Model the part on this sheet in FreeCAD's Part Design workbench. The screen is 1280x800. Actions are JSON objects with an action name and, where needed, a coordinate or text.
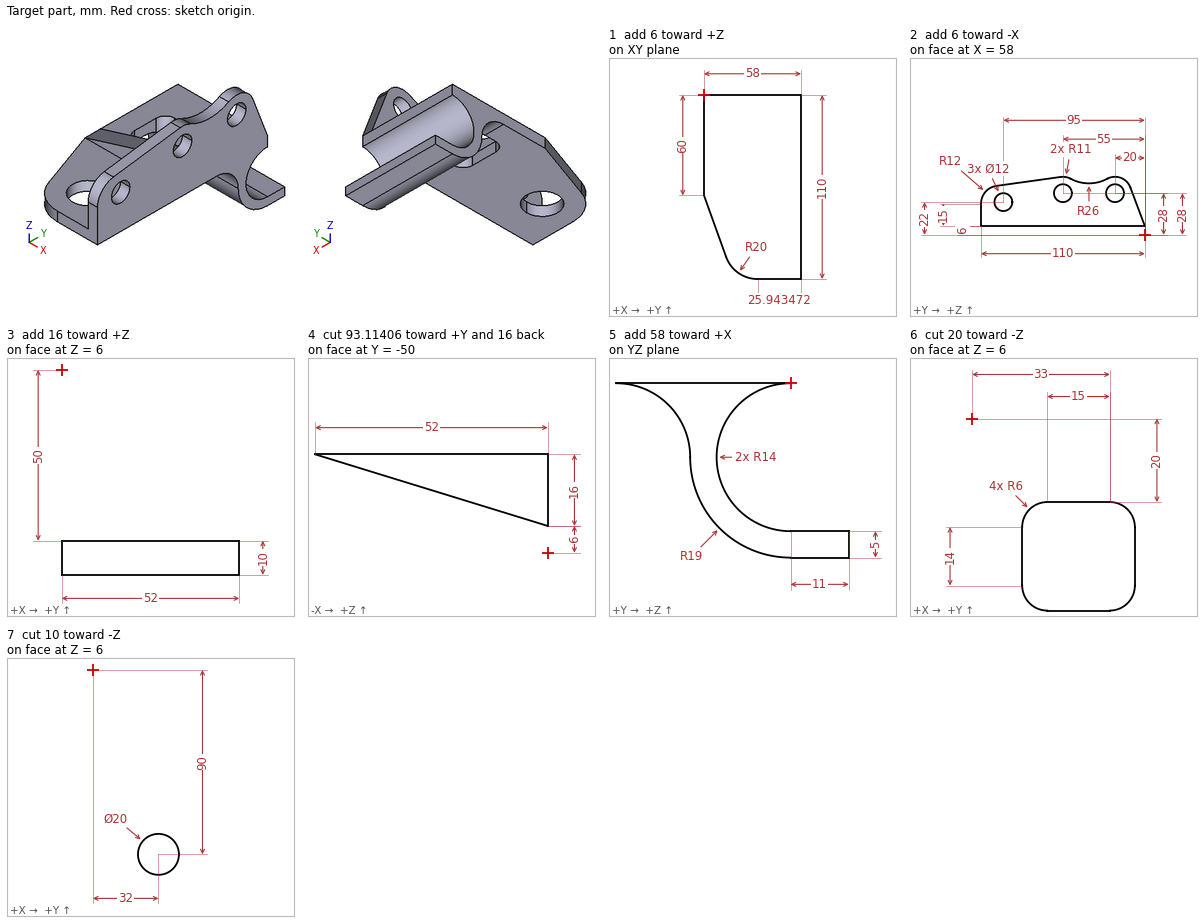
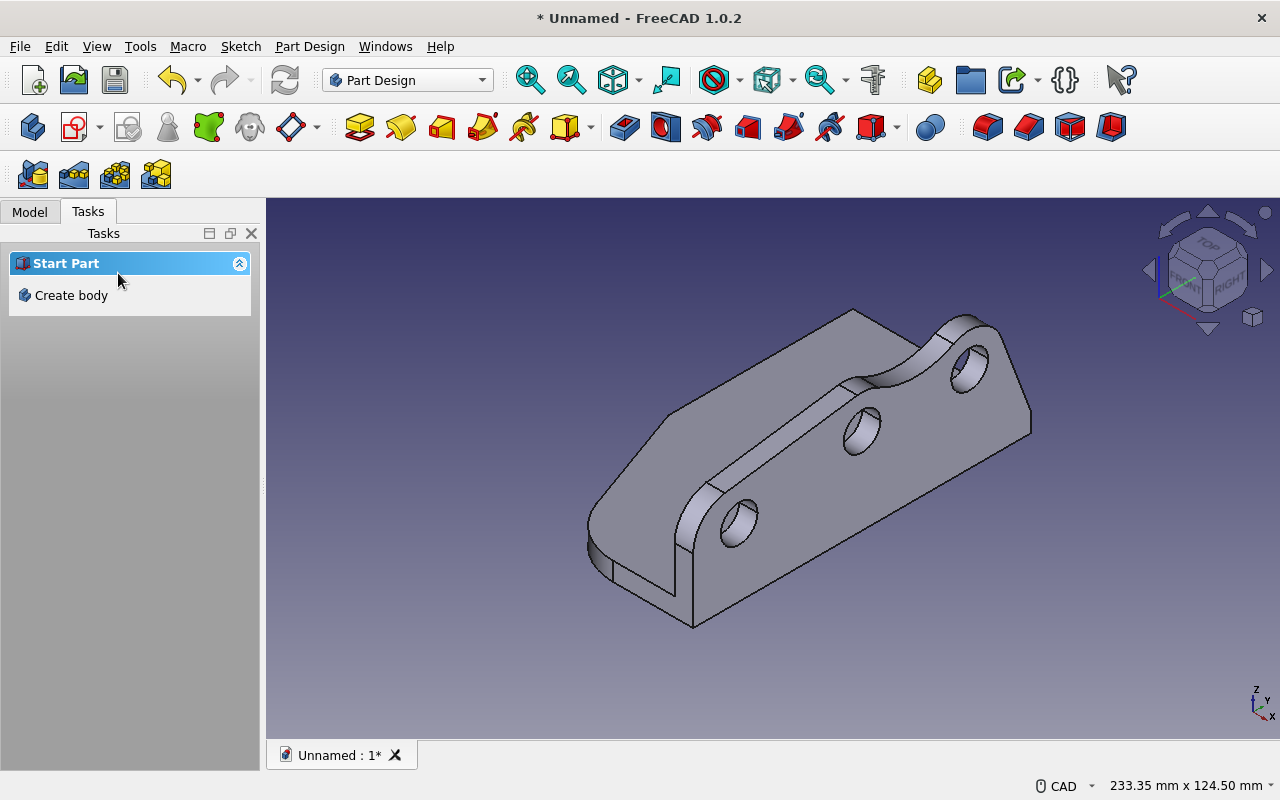
{"action": "left_click", "coordinate": [531, 80]}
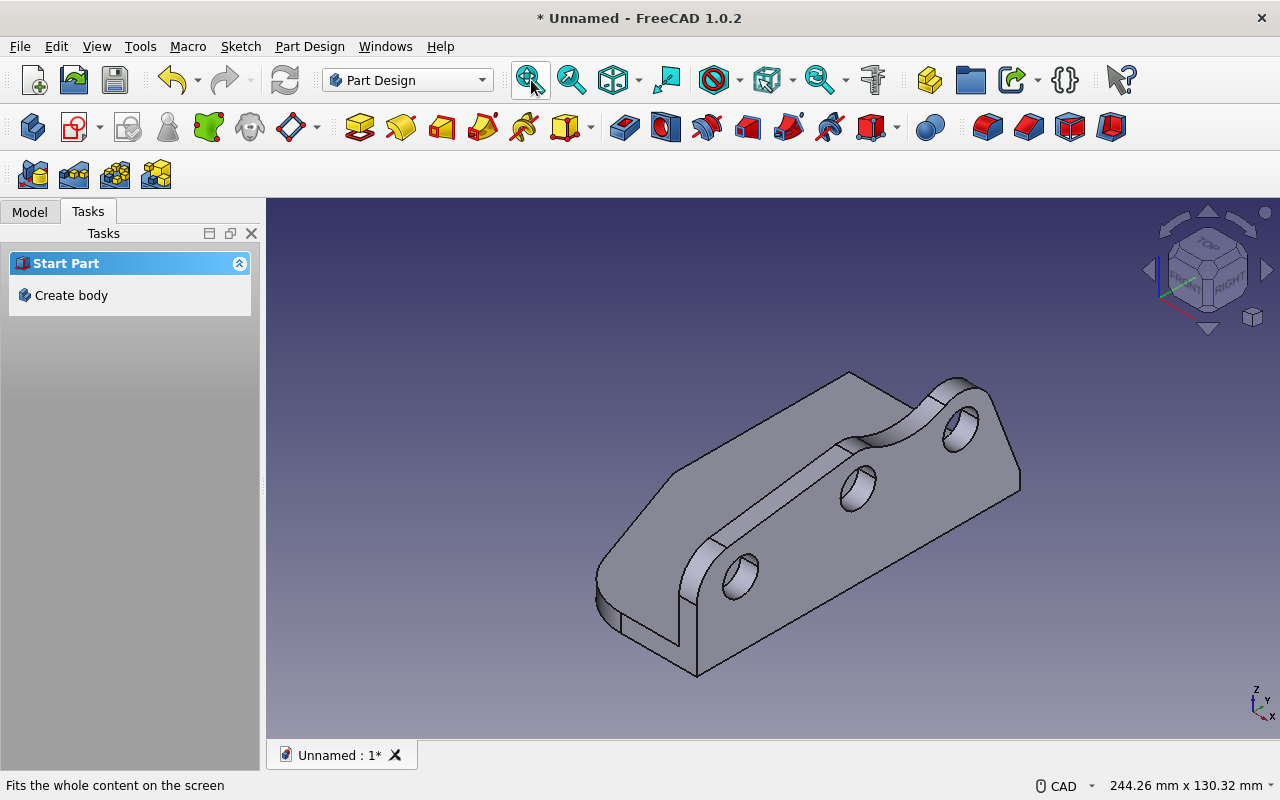
{"action": "left_click", "coordinate": [742, 496]}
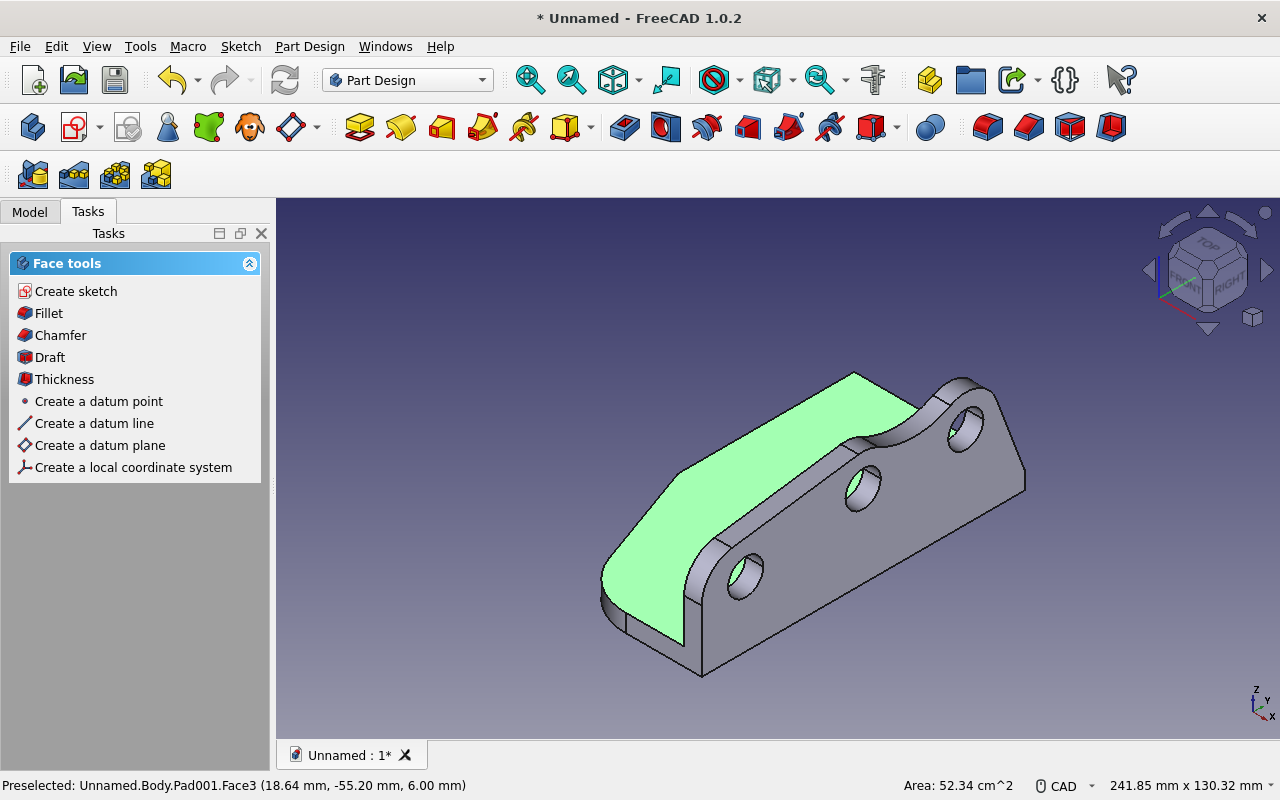
{"action": "left_click", "coordinate": [74, 128]}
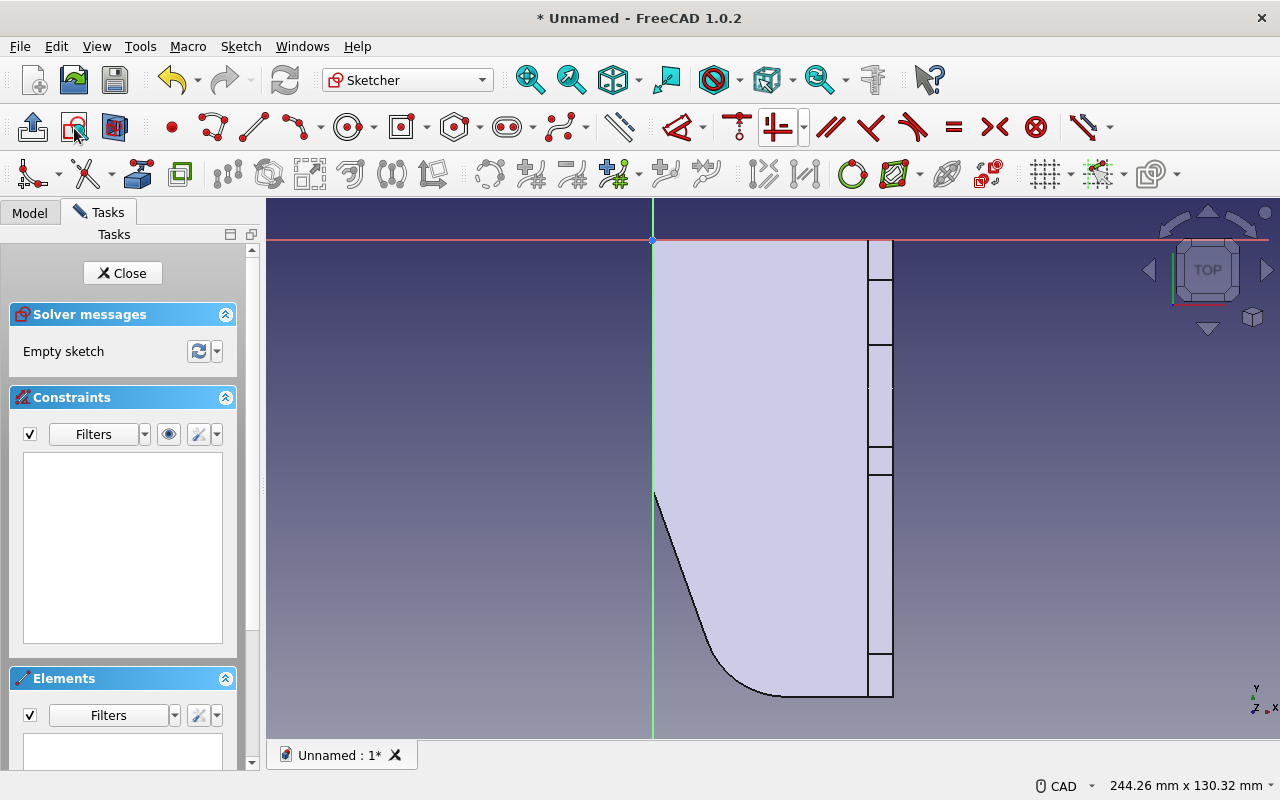
{"action": "scroll", "coordinate": [451, 711], "scroll_direction": "down", "scroll_amount": 1}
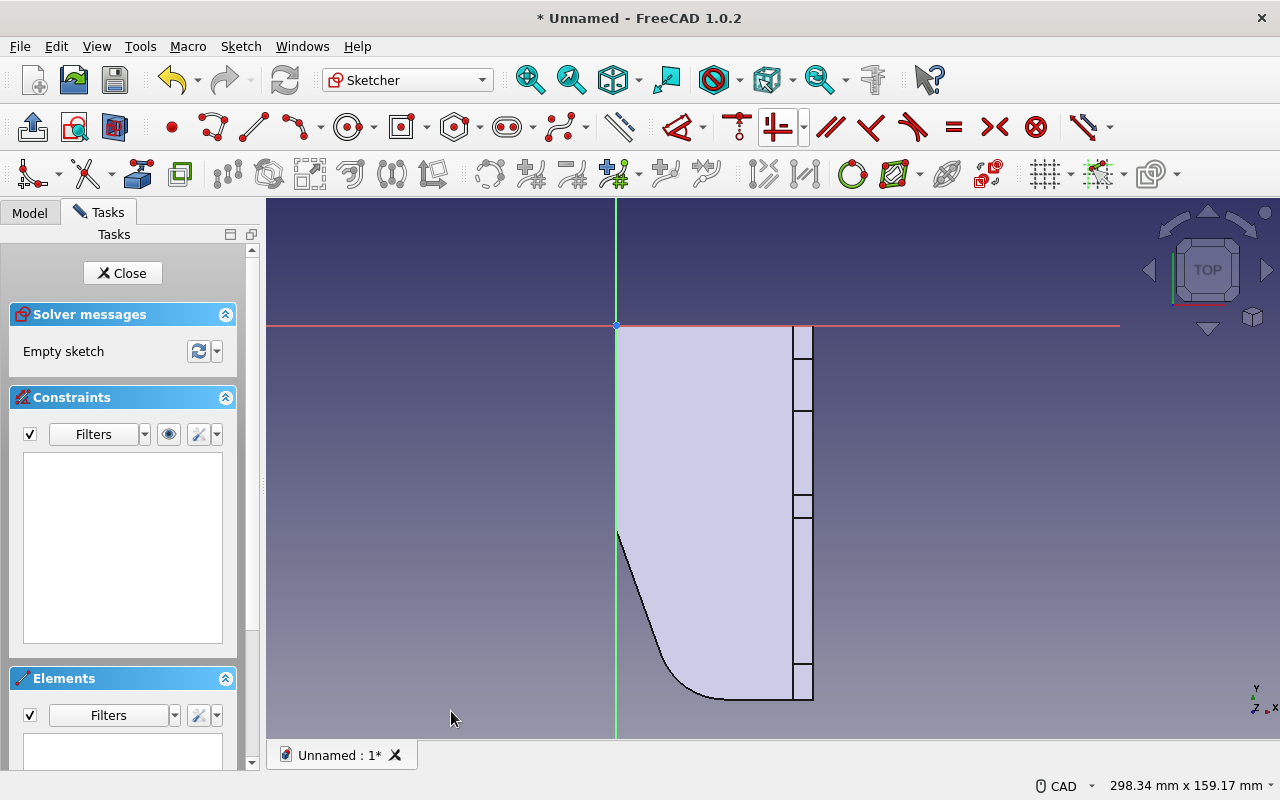
{"action": "scroll", "coordinate": [704, 378], "scroll_direction": "up", "scroll_amount": 3}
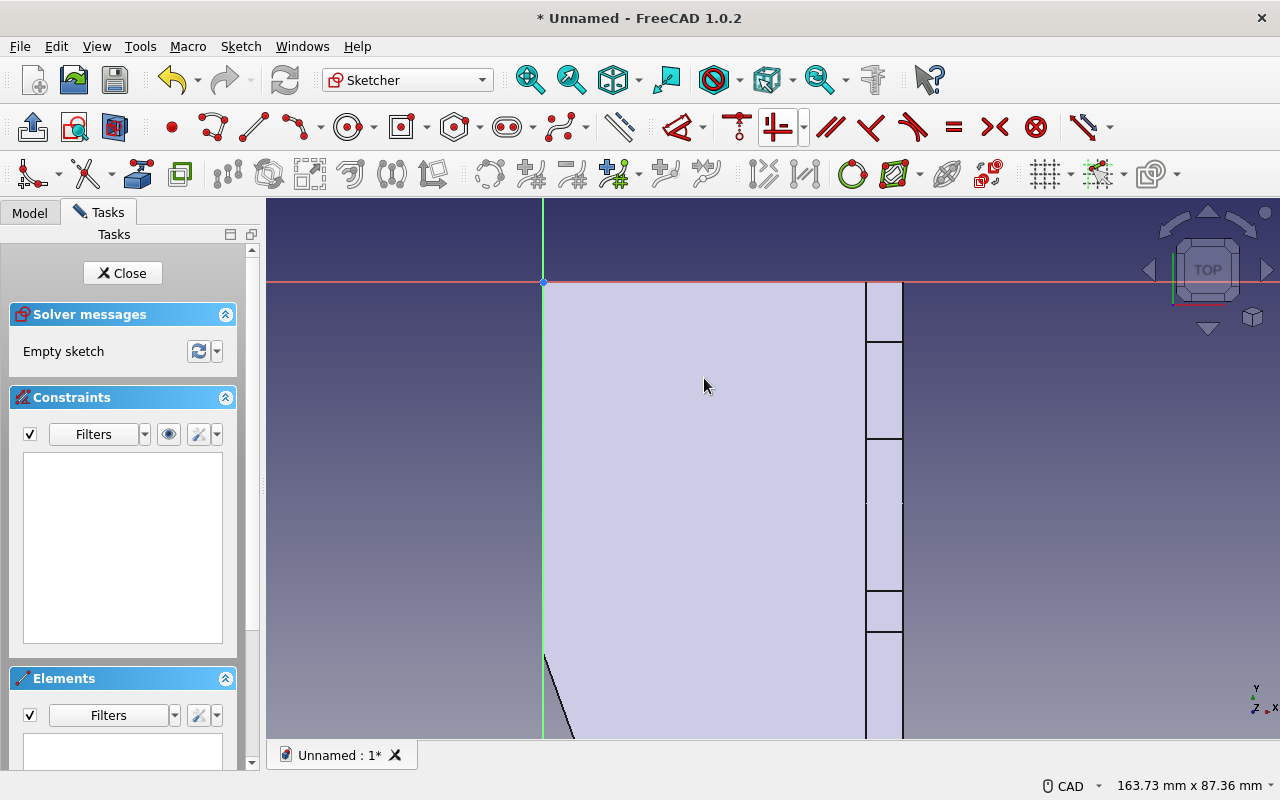
{"action": "key", "text": "g r"}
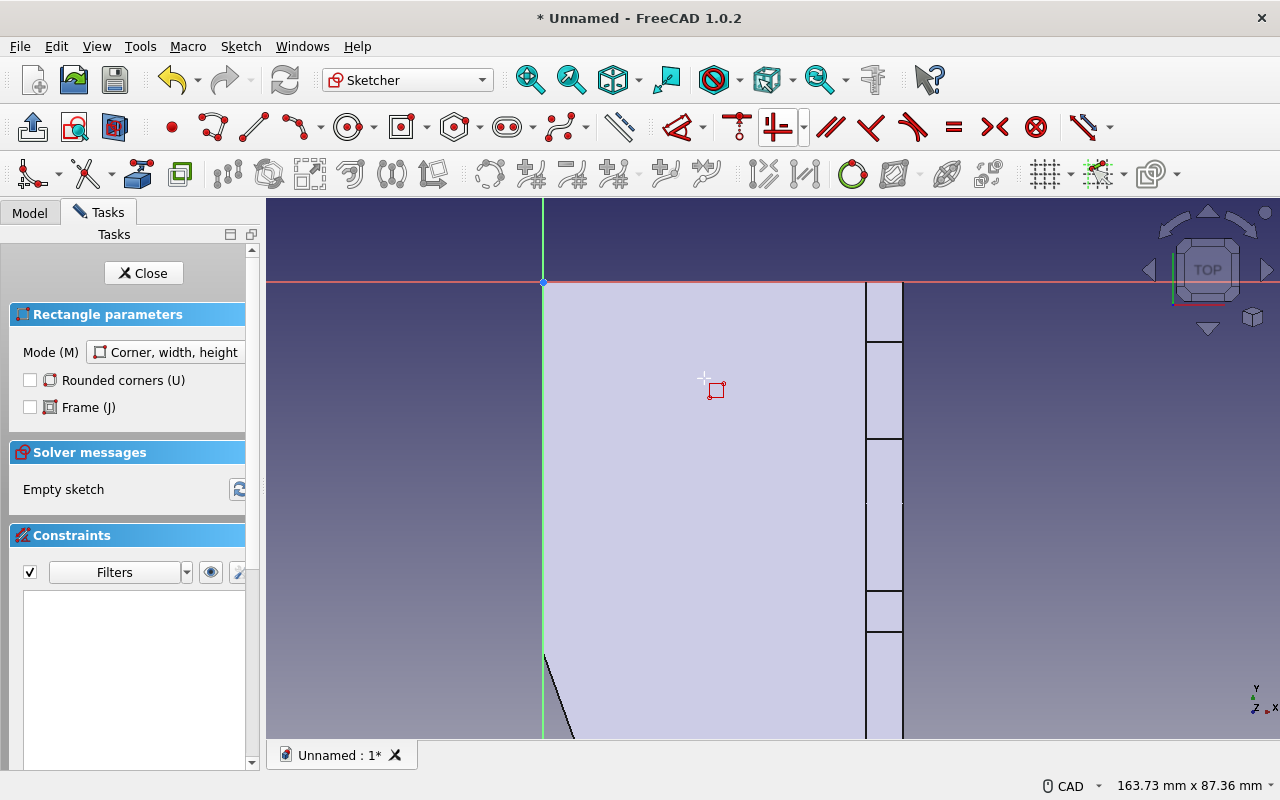
{"action": "left_click", "coordinate": [543, 592]}
{"action": "mouse_move", "coordinate": [866, 654]}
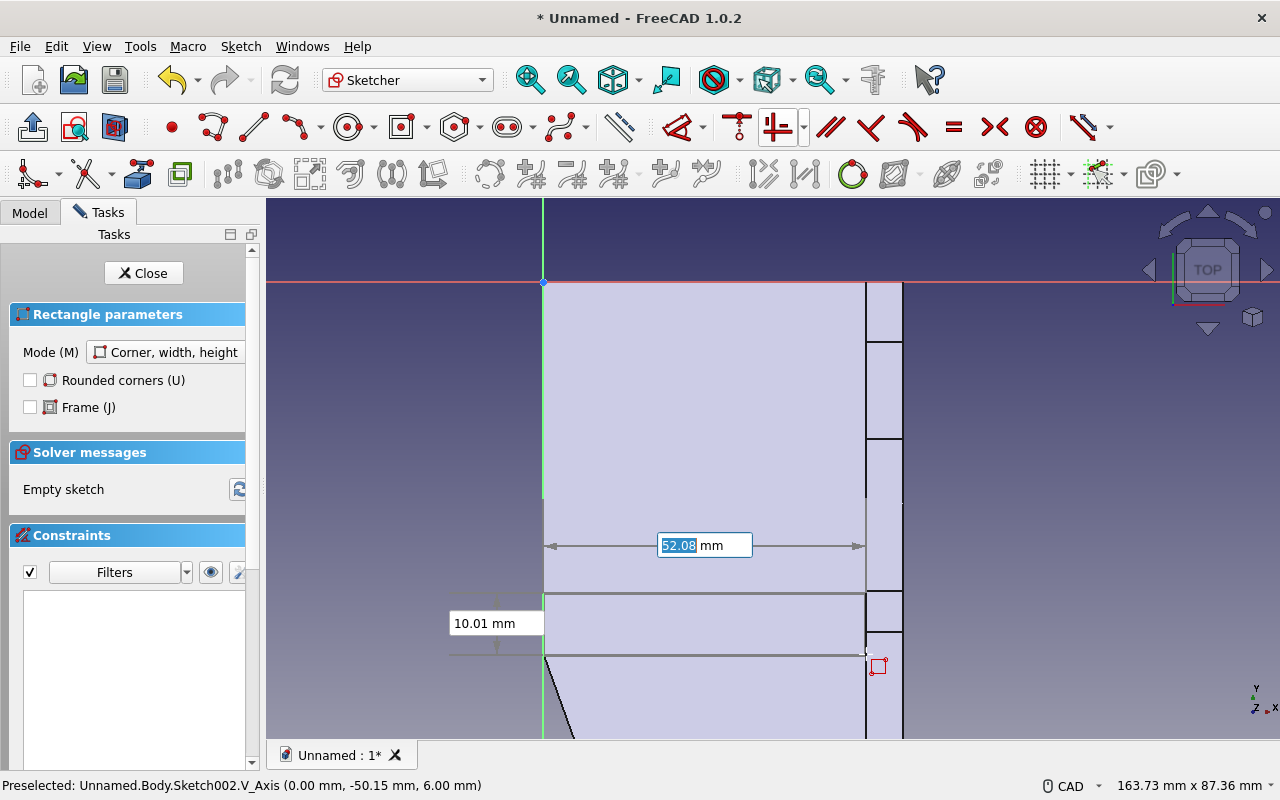
{"action": "type", "text": "52"}
{"action": "key", "text": "Tab"}
{"action": "type", "text": "10"}
{"action": "key", "text": "Return"}
{"action": "key", "text": "Escape"}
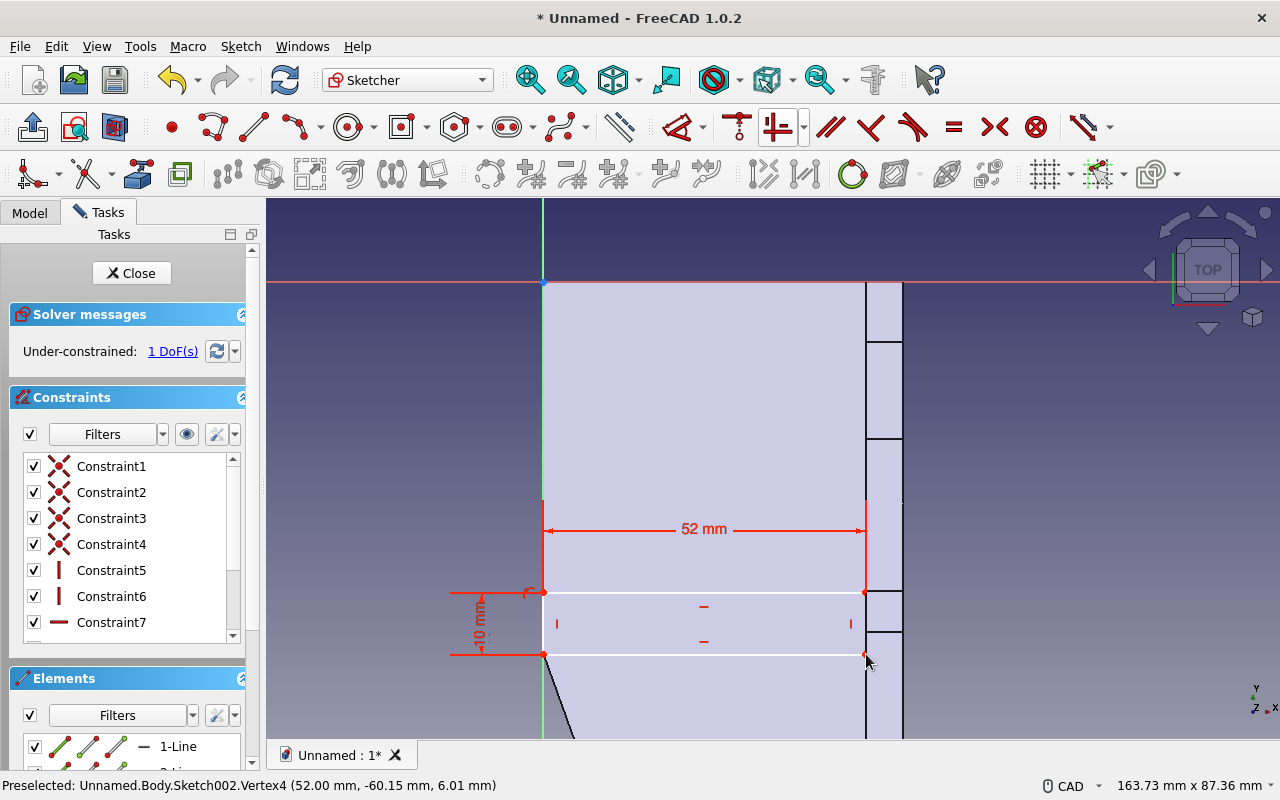
{"action": "left_click", "coordinate": [676, 128]}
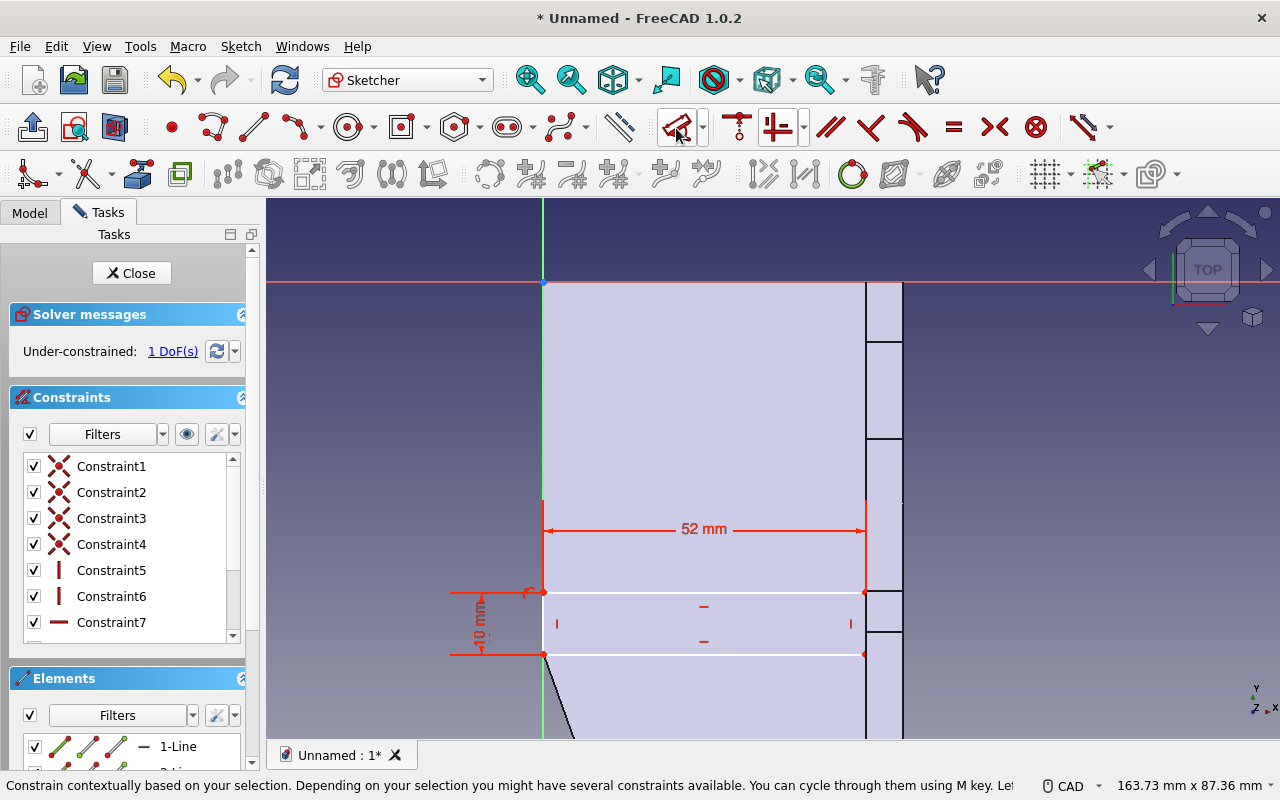
{"action": "left_click", "coordinate": [543, 593]}
{"action": "left_click", "coordinate": [509, 438]}